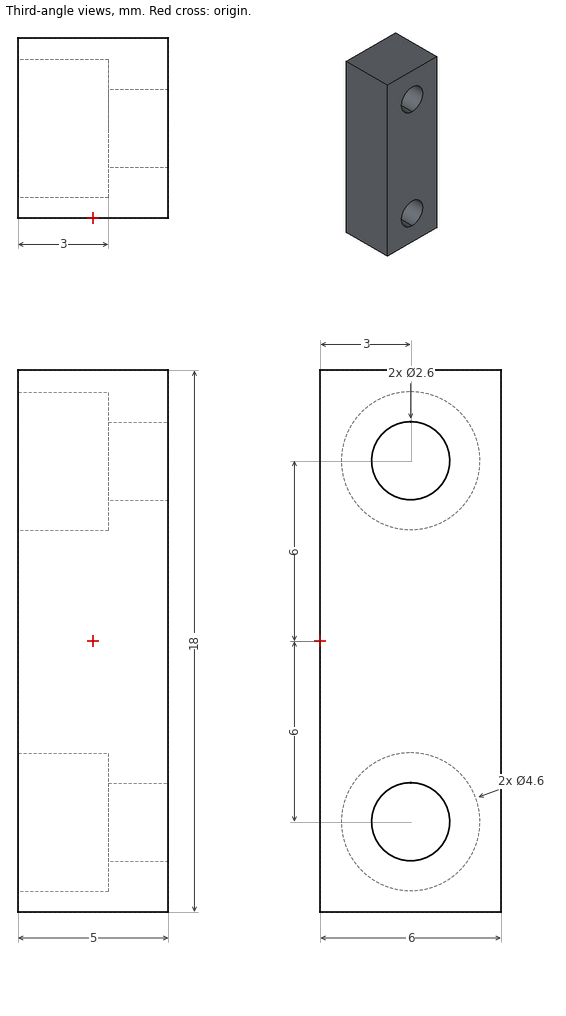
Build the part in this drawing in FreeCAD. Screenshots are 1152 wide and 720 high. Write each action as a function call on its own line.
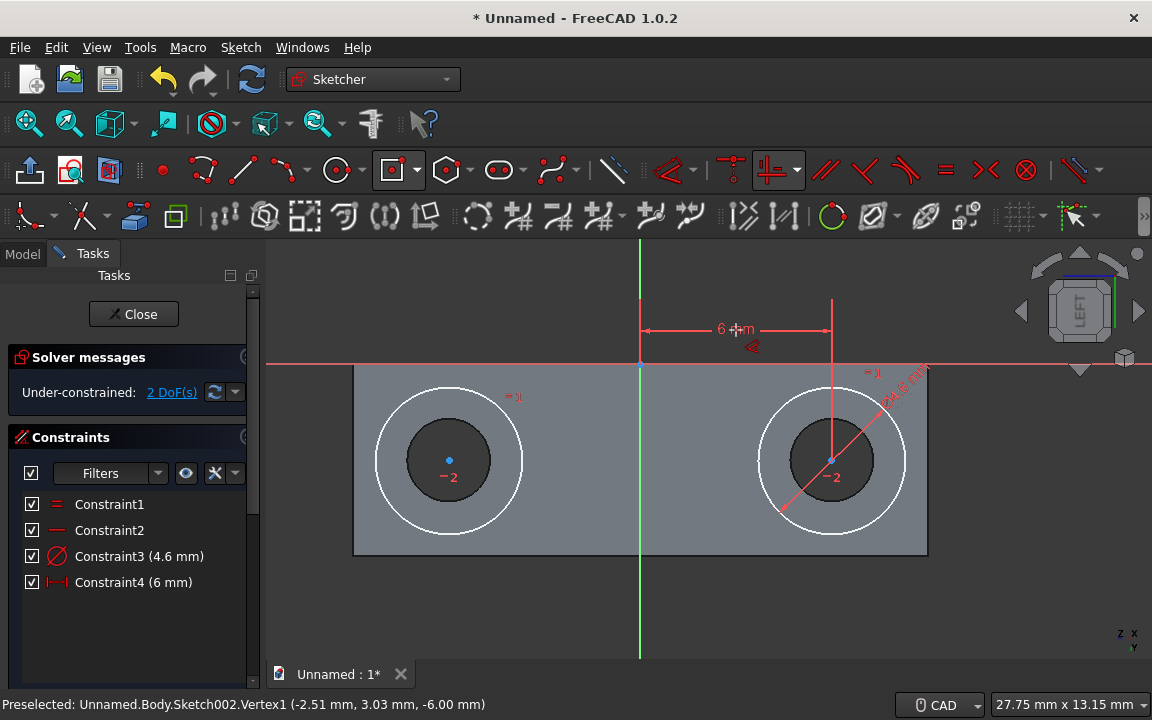
click(832, 461)
click(866, 413)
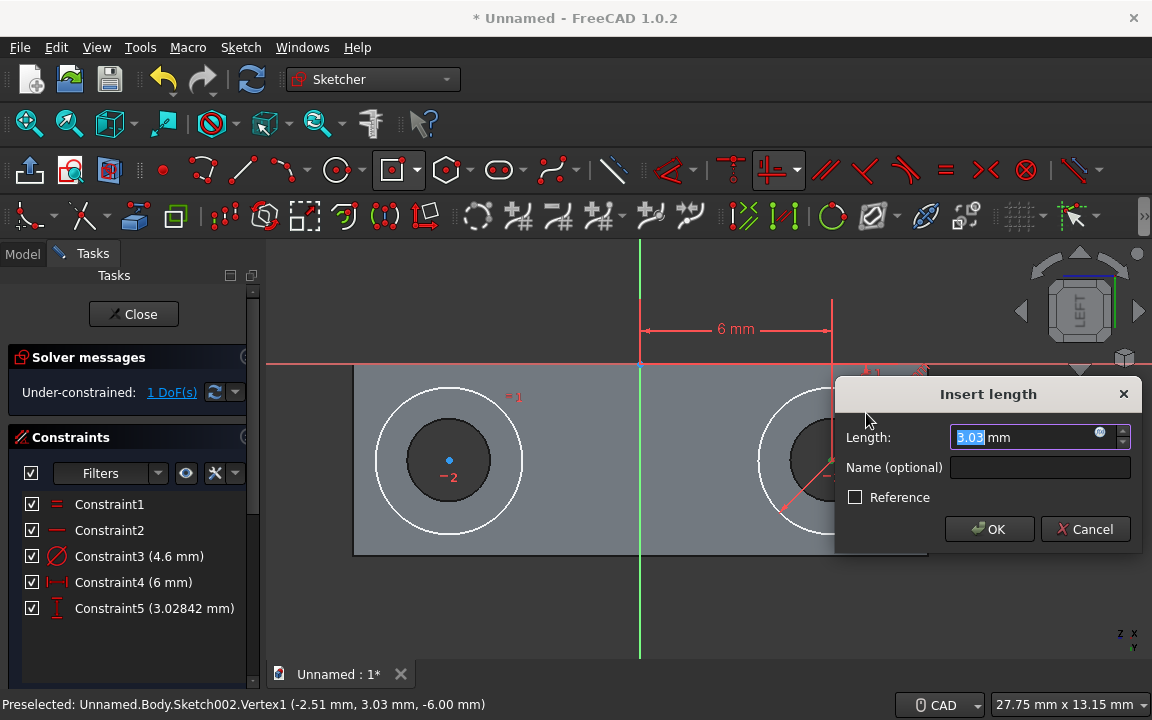
text(3)
key(Return)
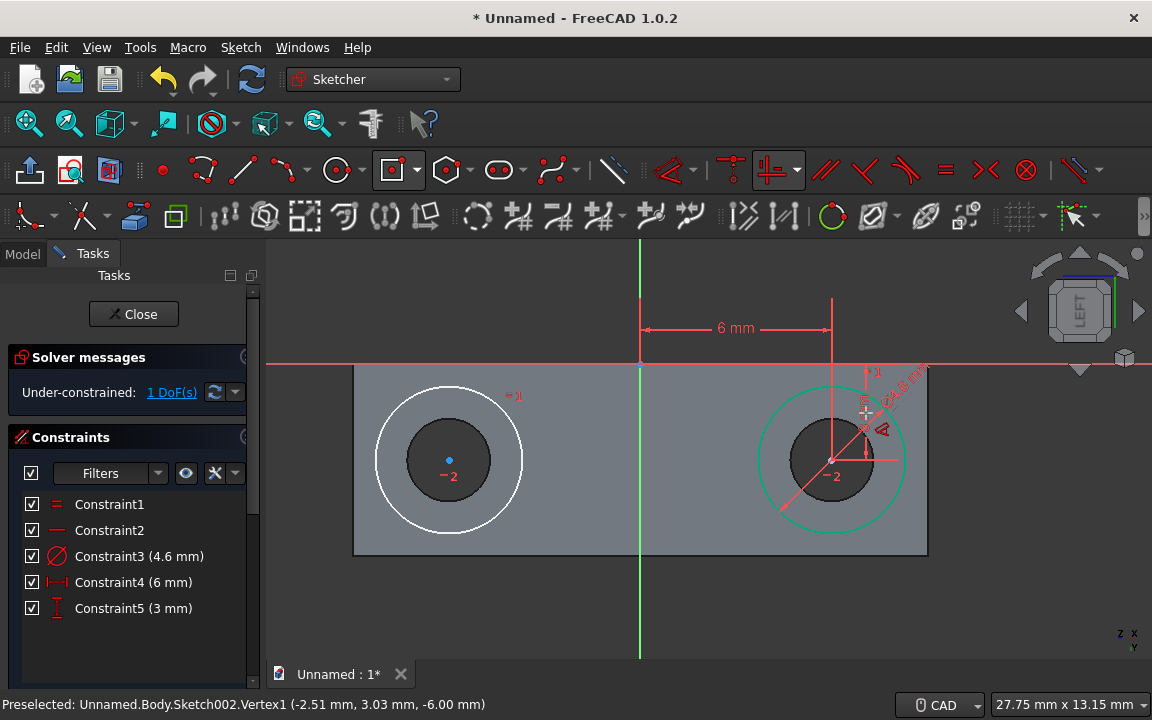
click(449, 460)
click(545, 330)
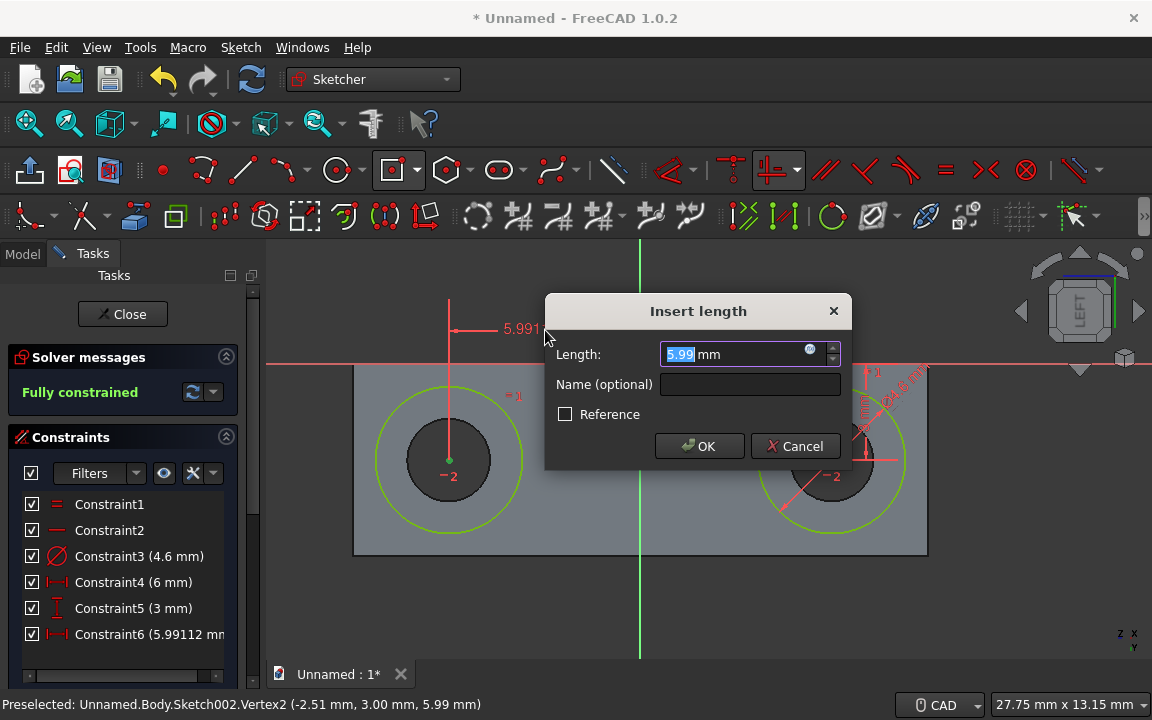
text(6)
key(Return)
key(Escape)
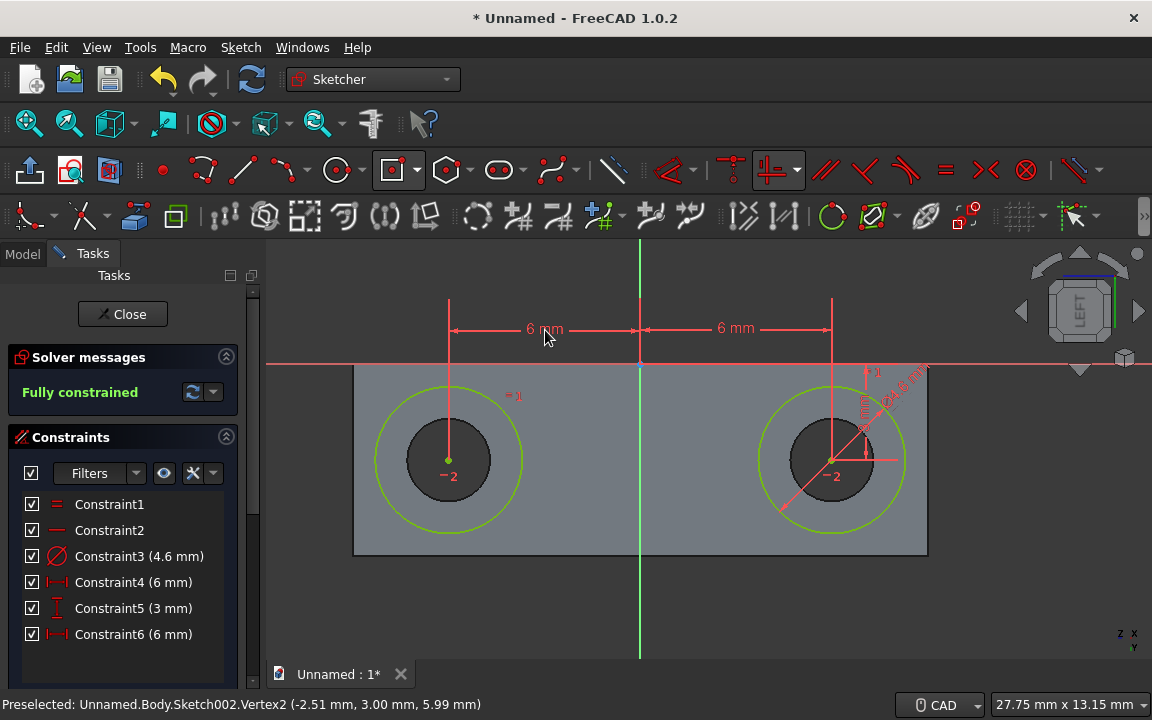
click(123, 314)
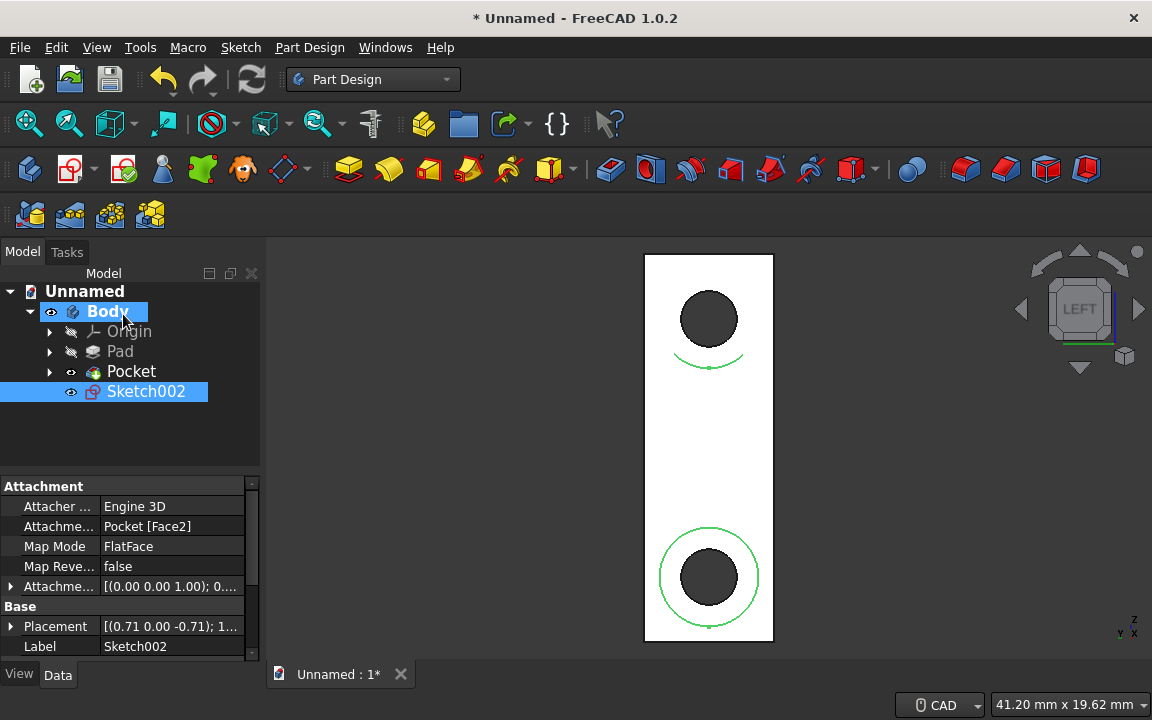
click(612, 170)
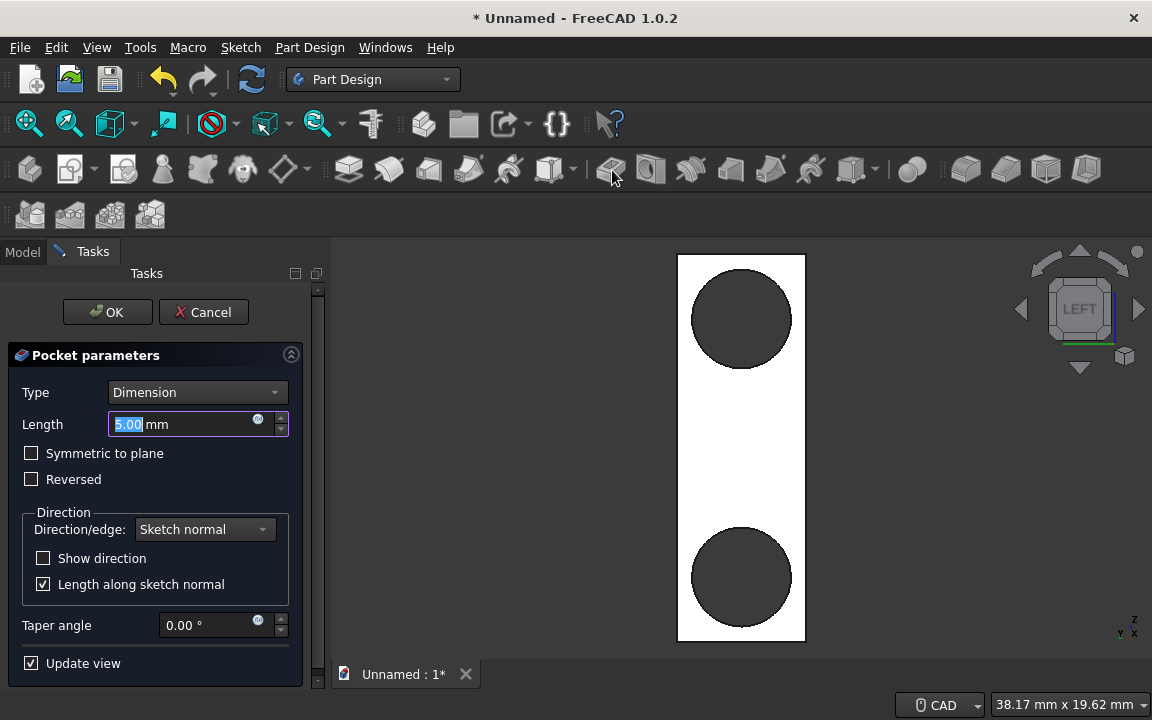
text(3)
key(Tab)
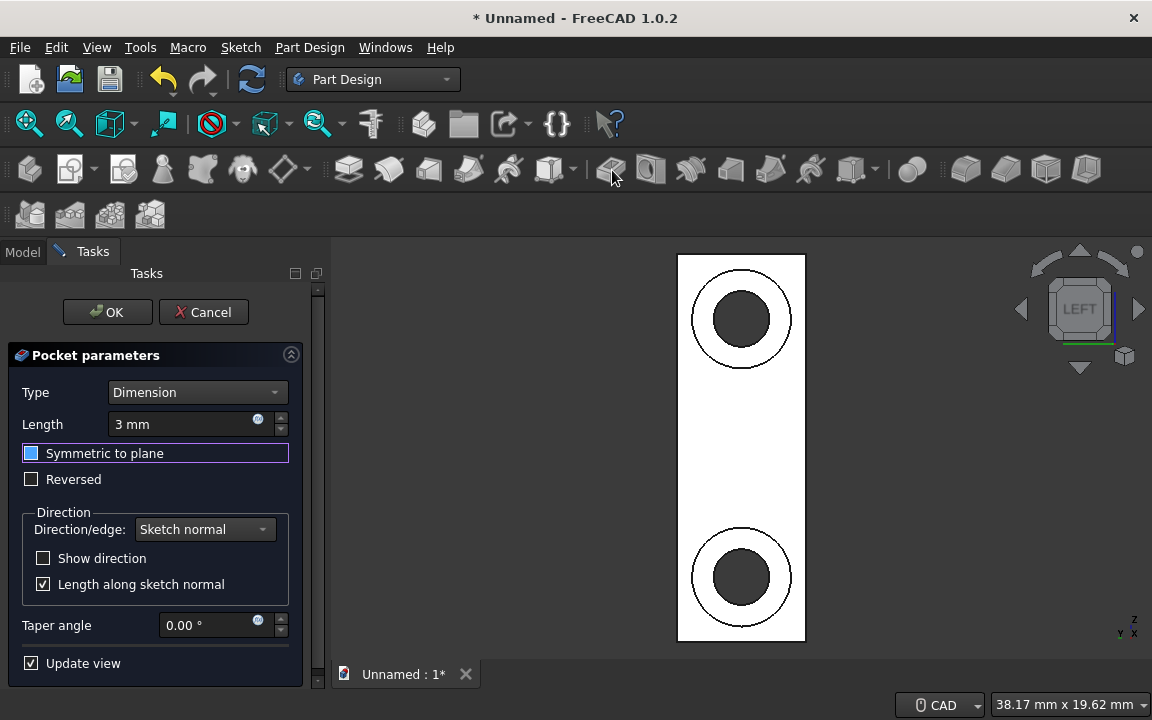
click(108, 312)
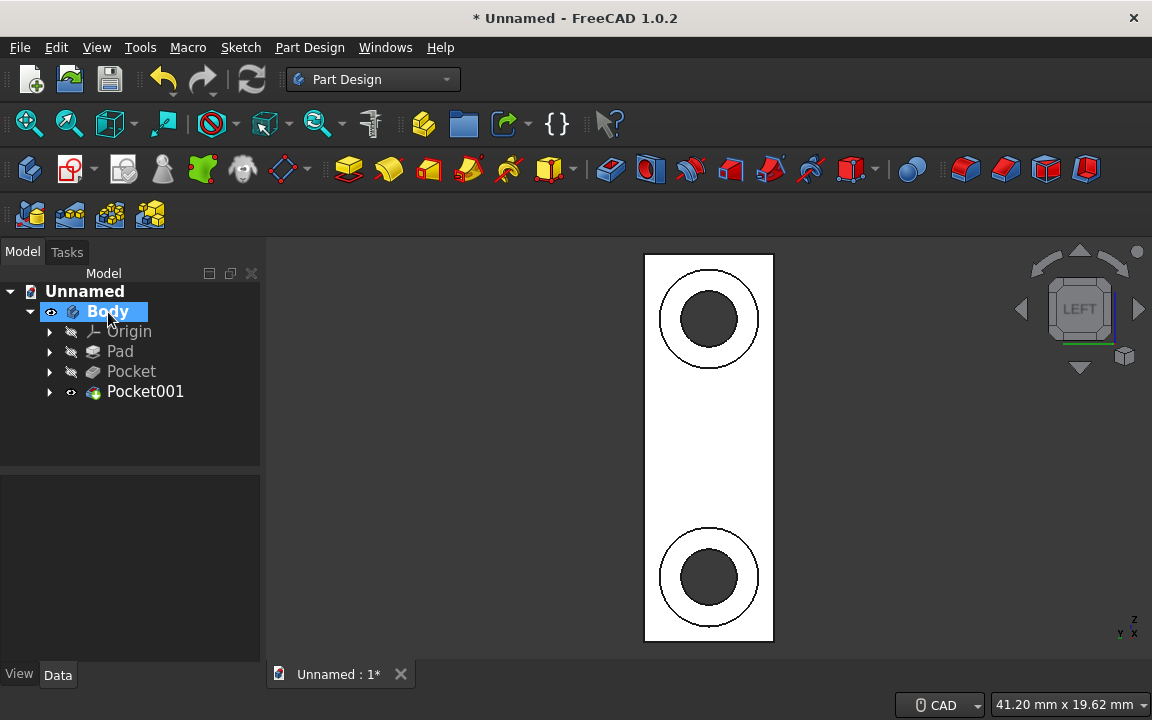
key(0)